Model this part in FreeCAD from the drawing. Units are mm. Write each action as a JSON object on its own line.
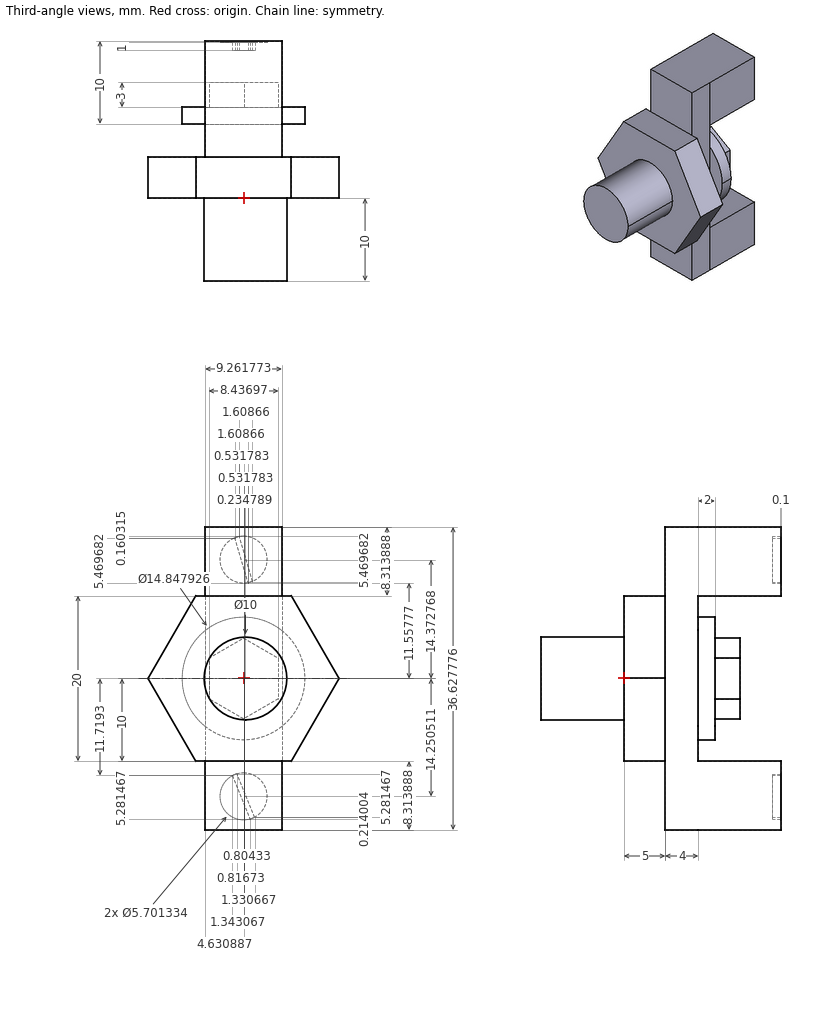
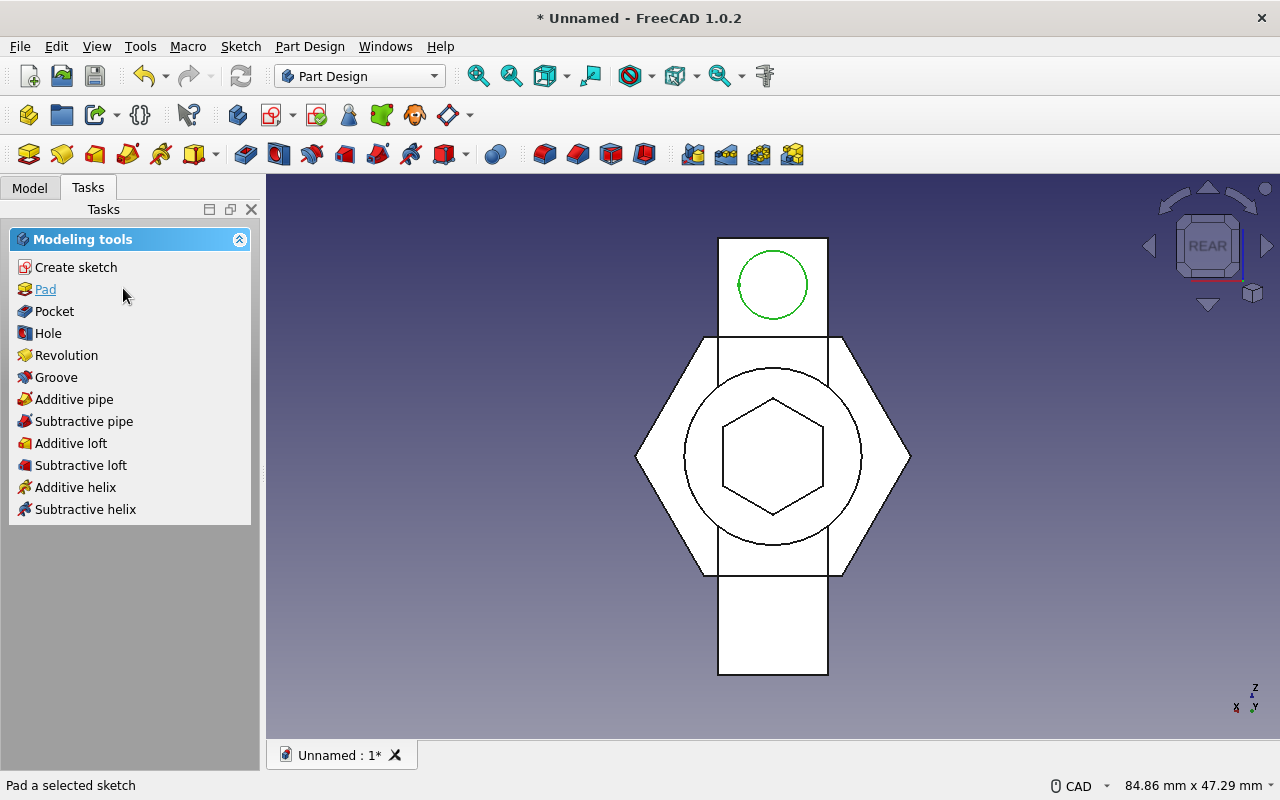
{"action": "left_click", "coordinate": [246, 154]}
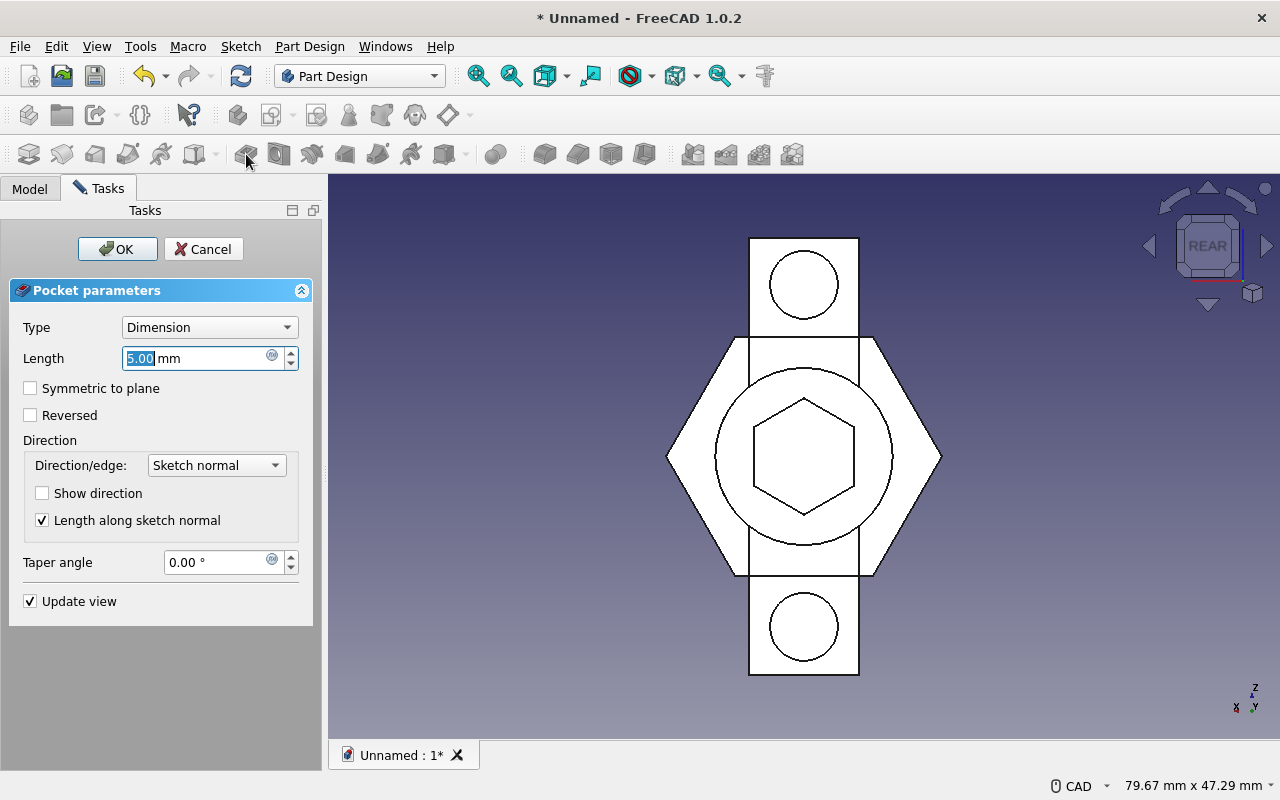
{"action": "type", "text": "0.1"}
{"action": "key", "text": "Tab"}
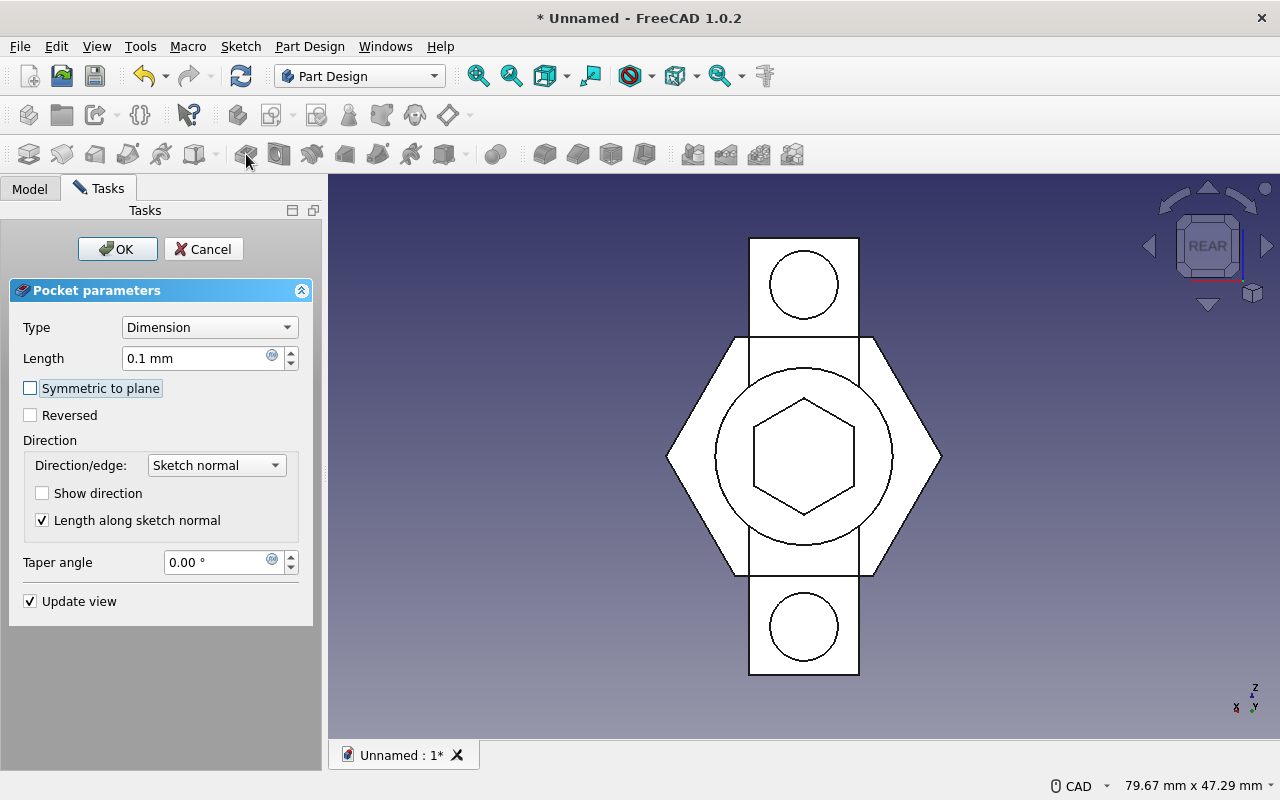
{"action": "left_click", "coordinate": [118, 249]}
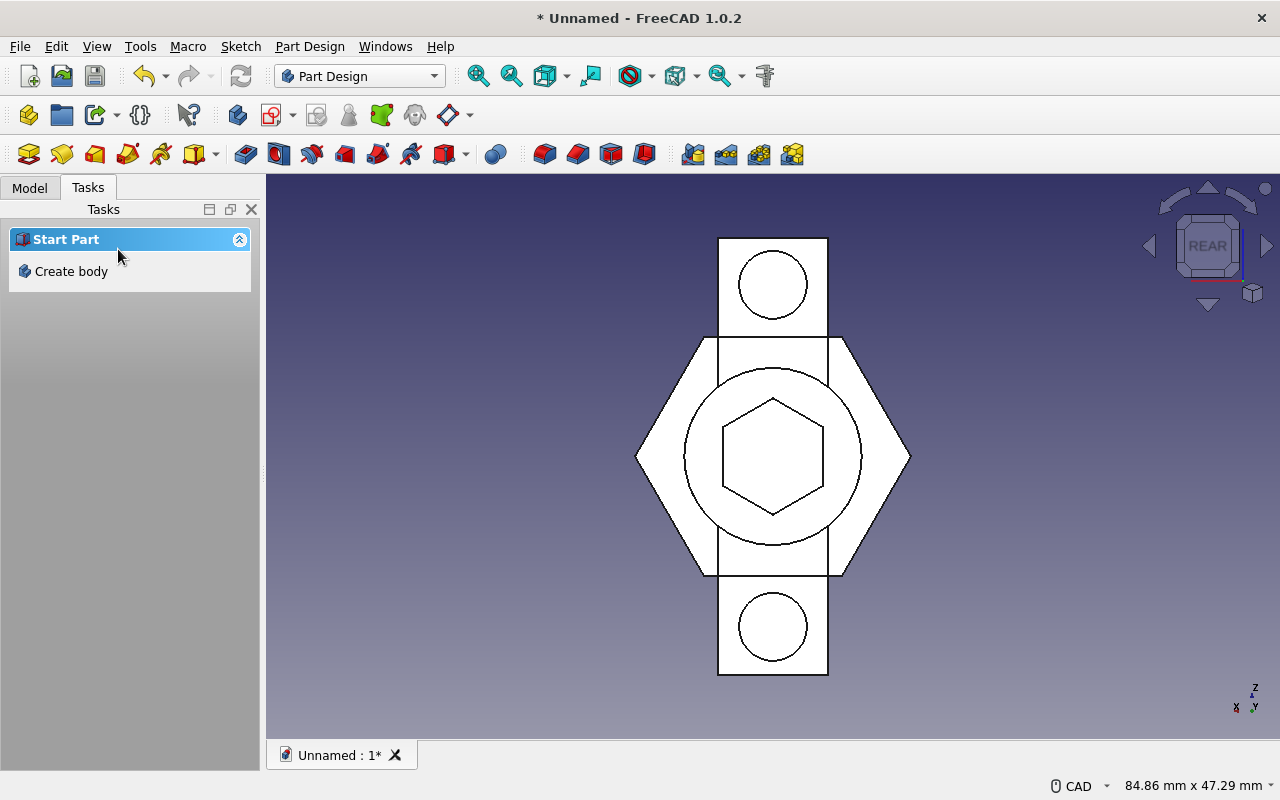
{"action": "left_click", "coordinate": [773, 284]}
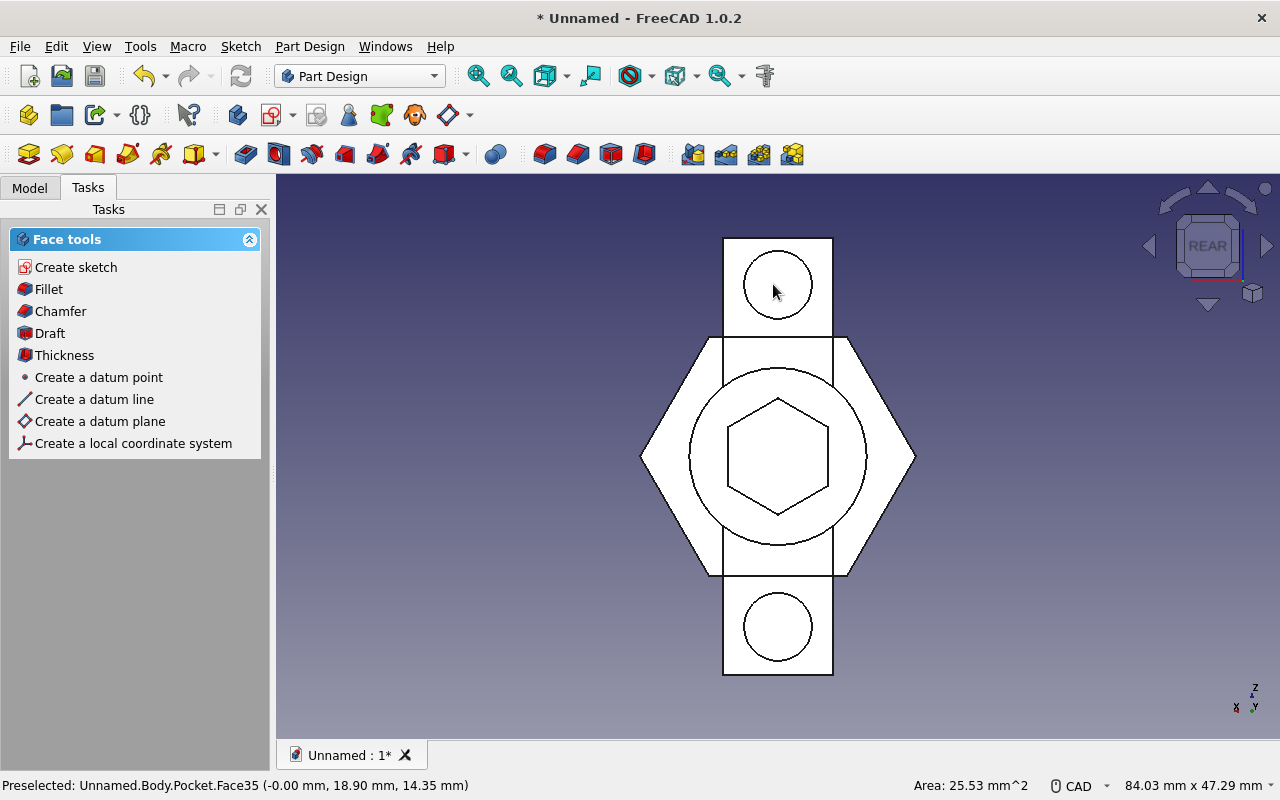
{"action": "left_click", "coordinate": [270, 116]}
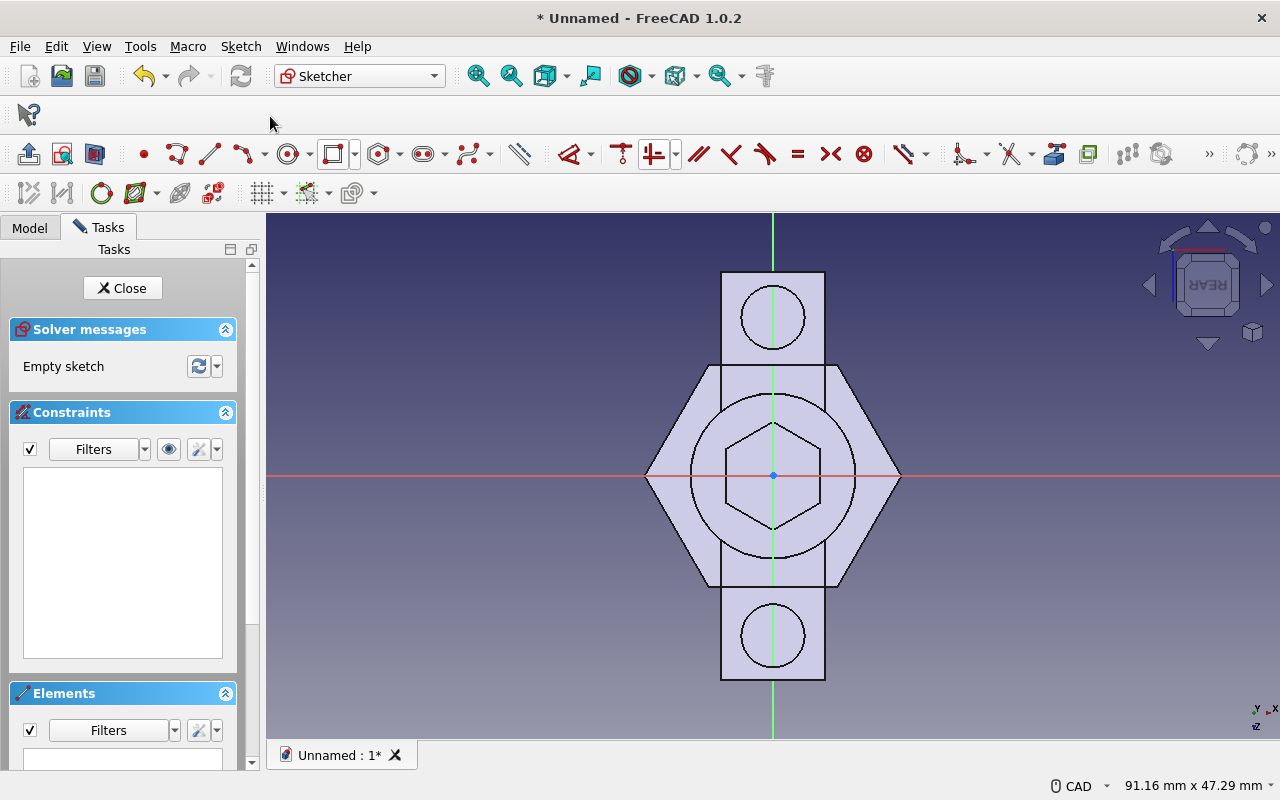
{"action": "left_click", "coordinate": [177, 154]}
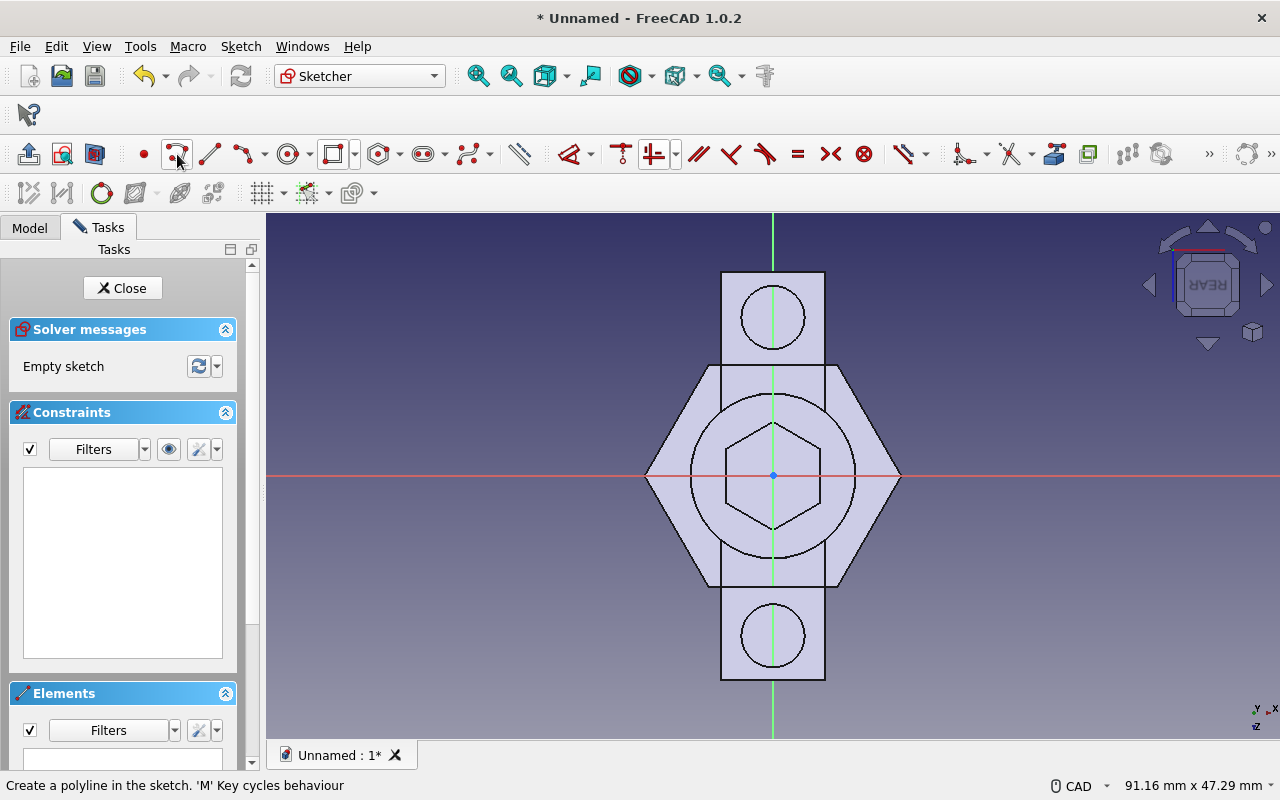
{"action": "scroll", "coordinate": [764, 348], "scroll_direction": "up", "scroll_amount": 3}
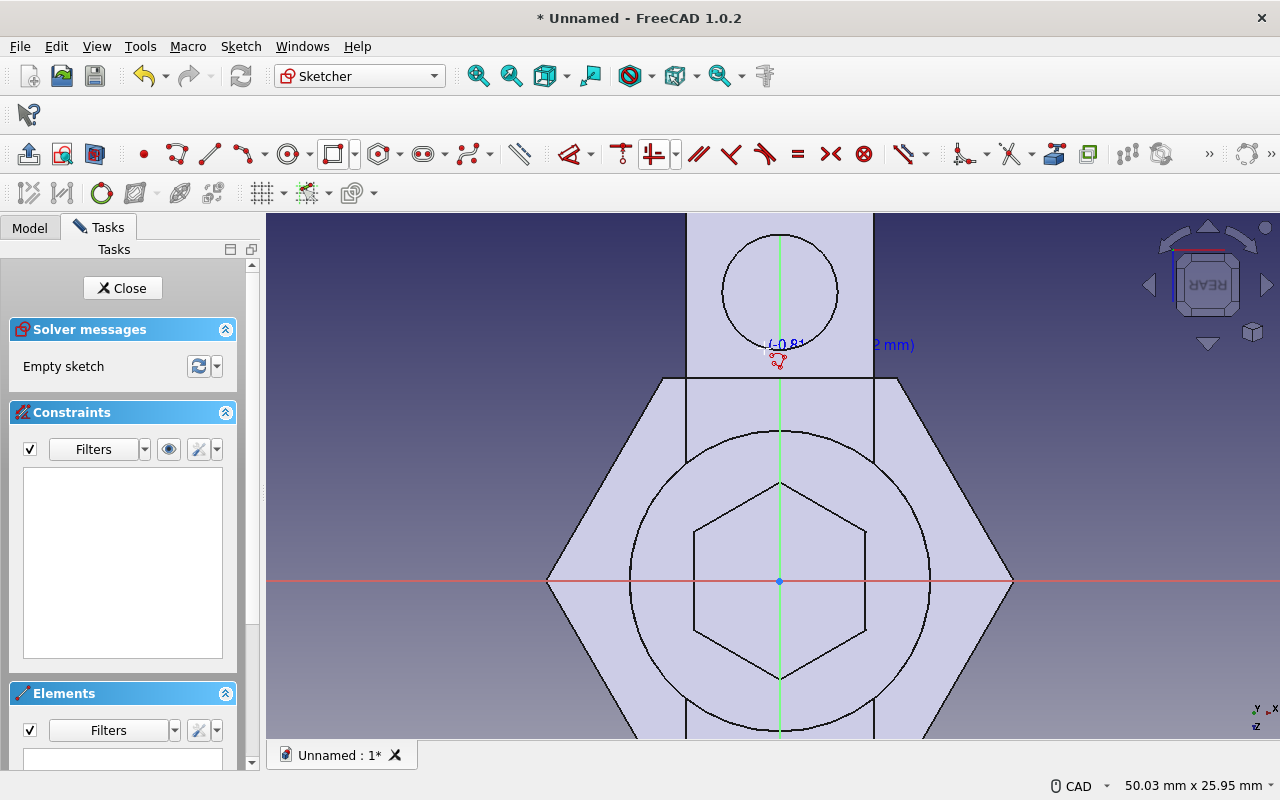
{"action": "left_click", "coordinate": [763, 348]}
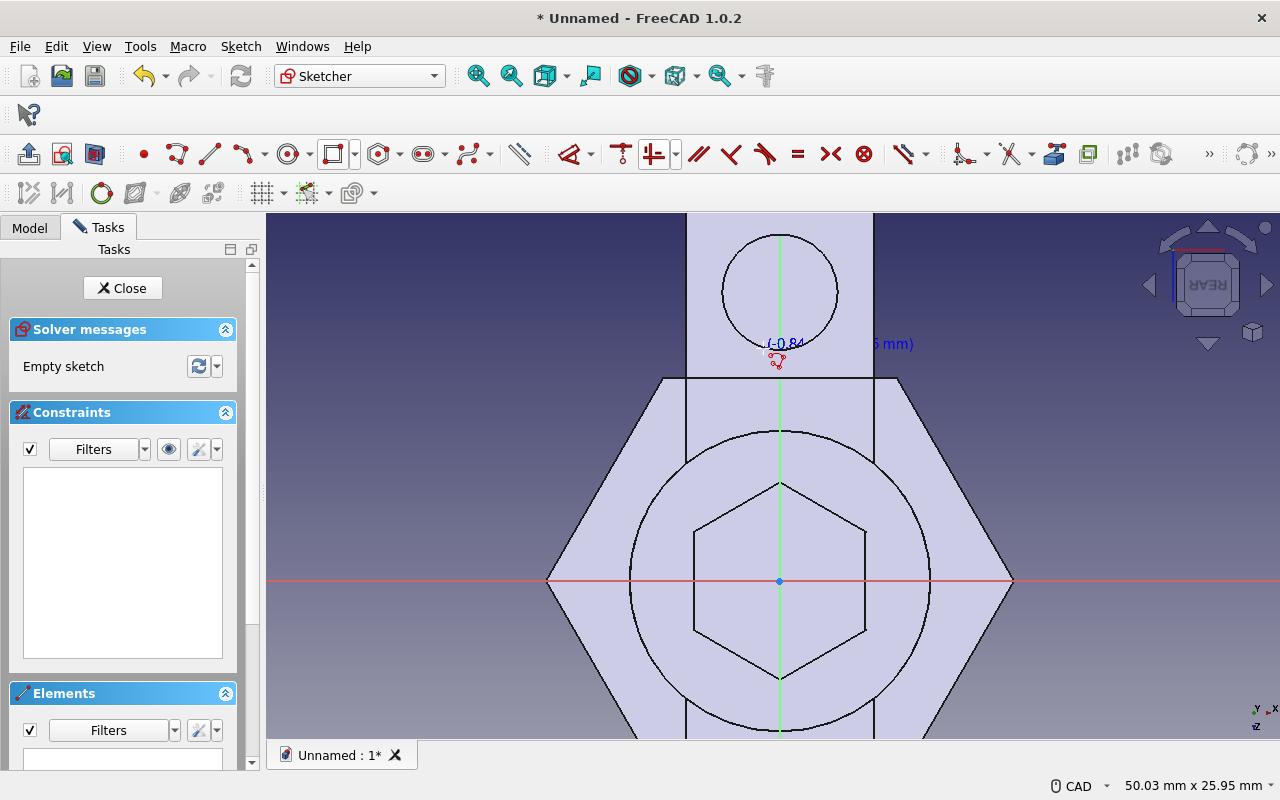
{"action": "scroll", "coordinate": [643, 389], "scroll_direction": "down", "scroll_amount": 4}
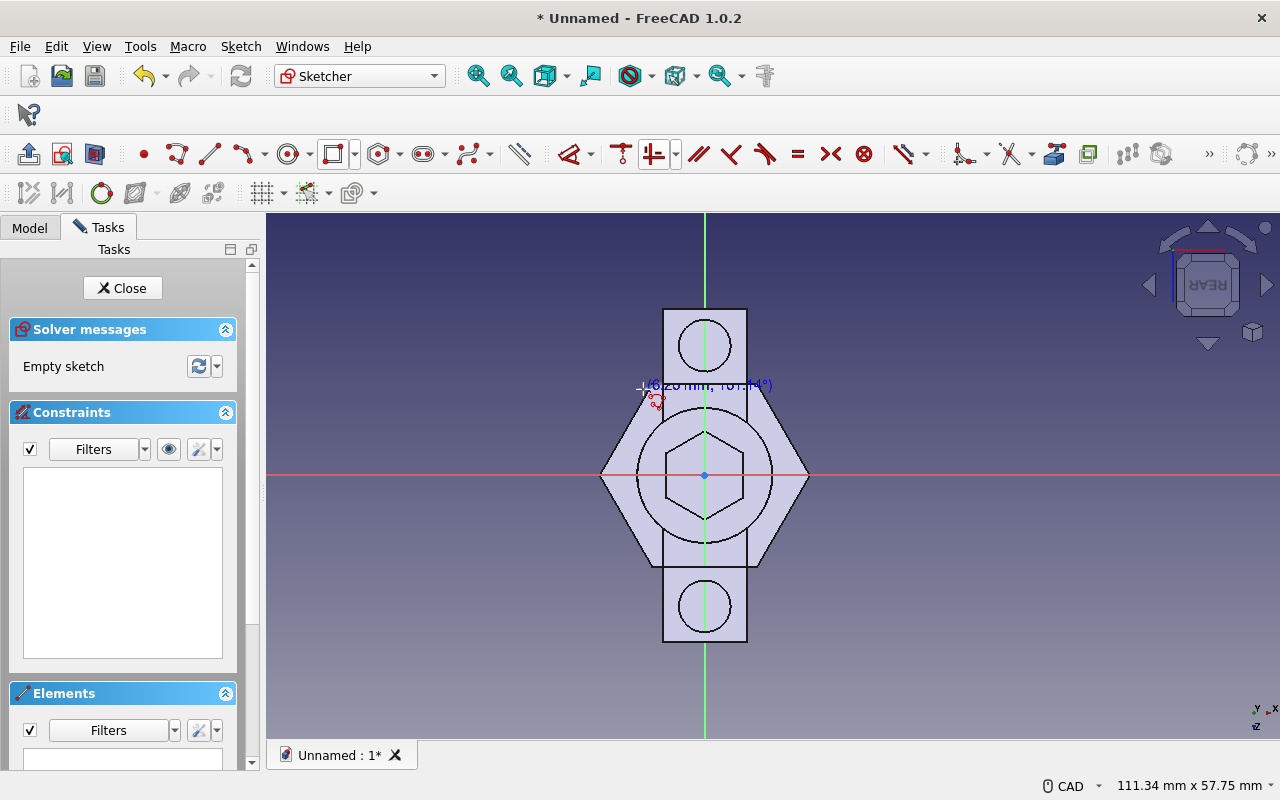
{"action": "scroll", "coordinate": [717, 323], "scroll_direction": "up", "scroll_amount": 2}